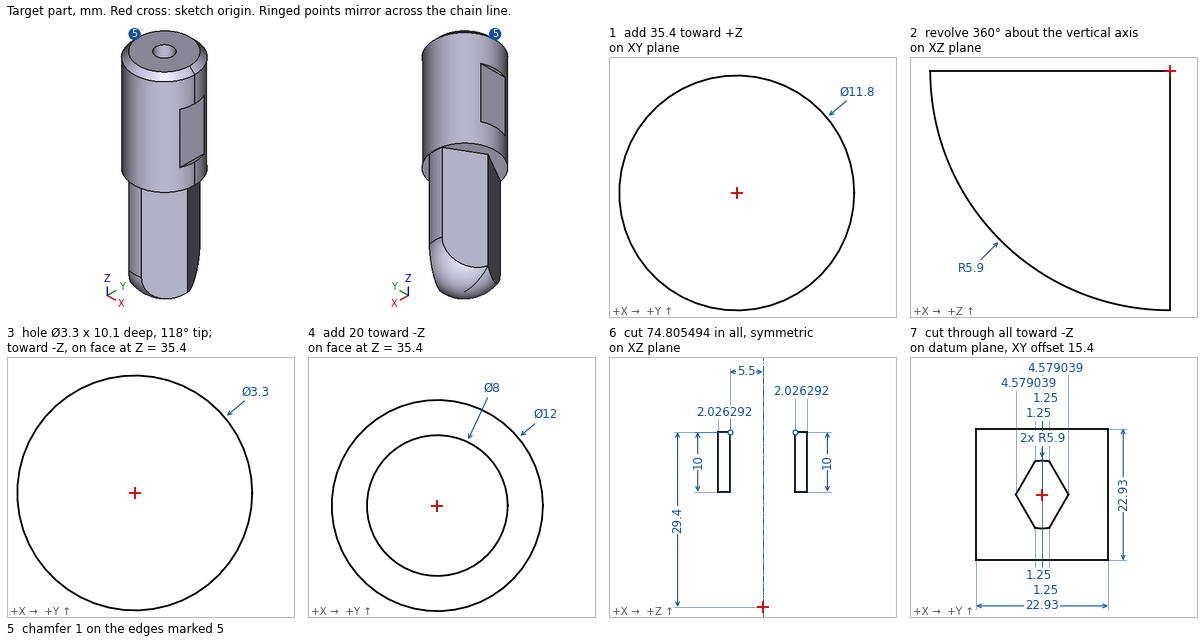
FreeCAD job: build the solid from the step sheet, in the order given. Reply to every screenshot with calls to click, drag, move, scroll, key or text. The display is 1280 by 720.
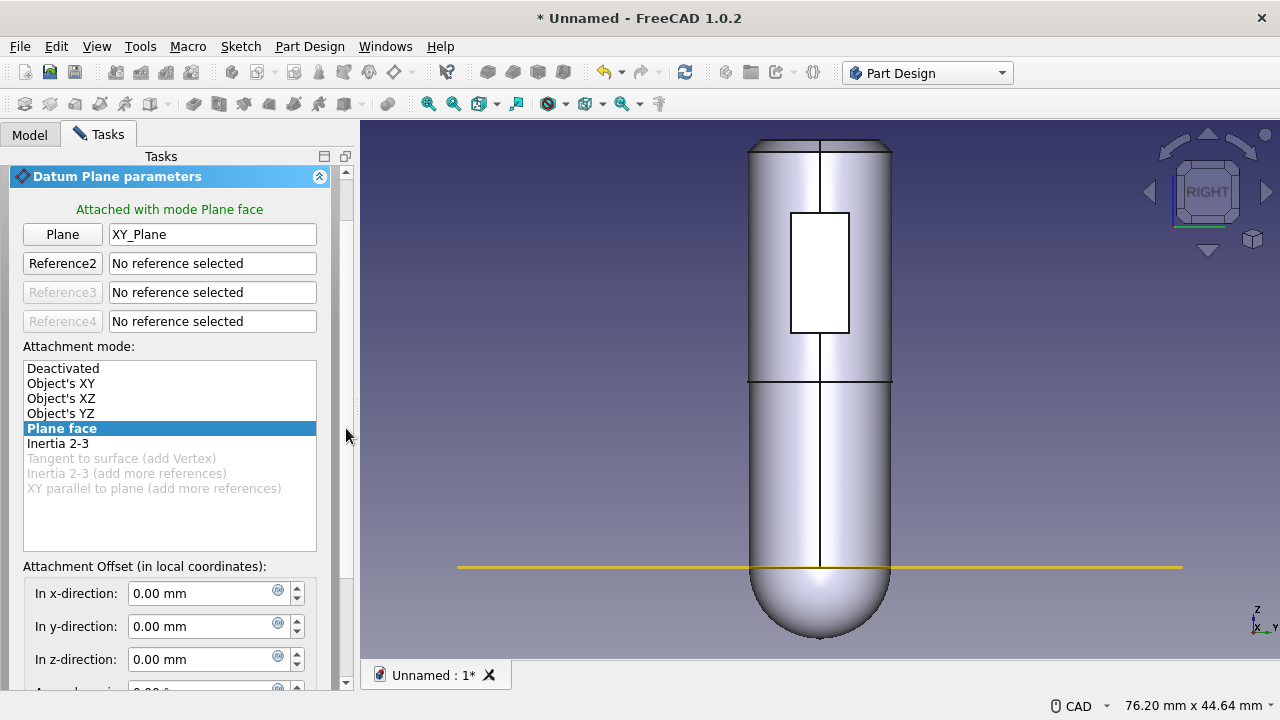
triple_click(210, 600)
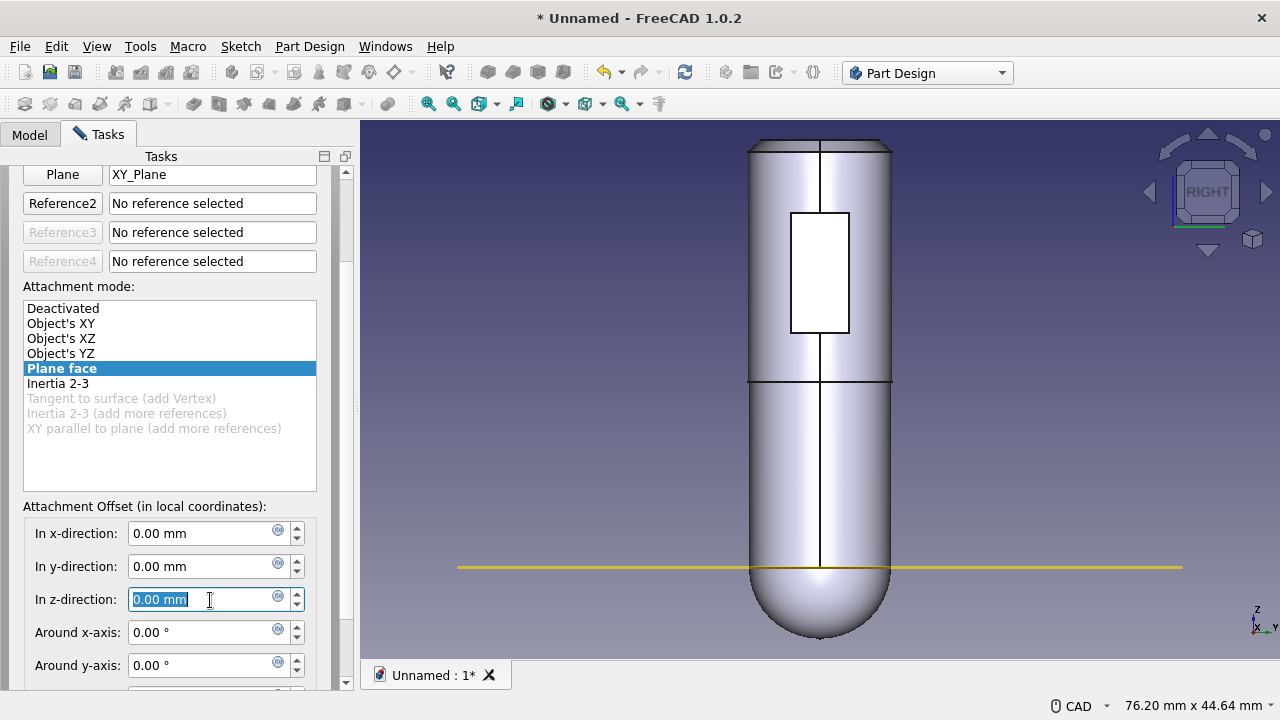
text(15.4)
key(Tab)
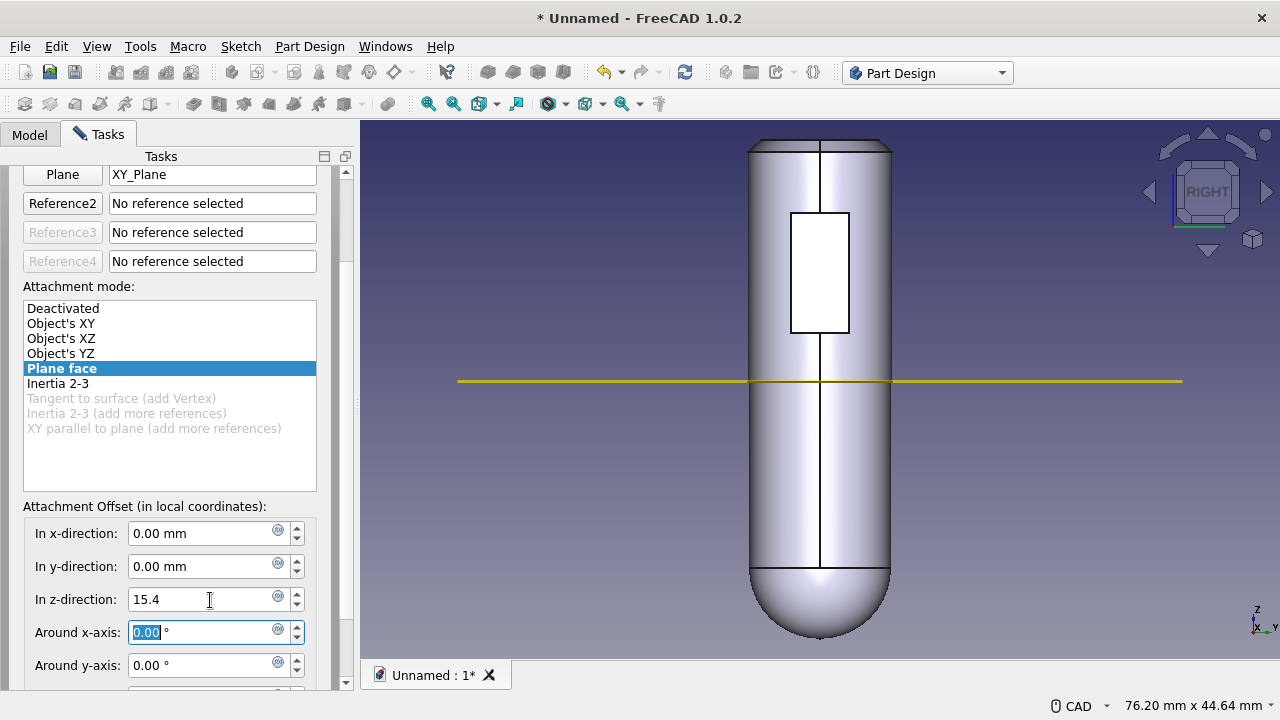
scroll(346, 428, up, 3)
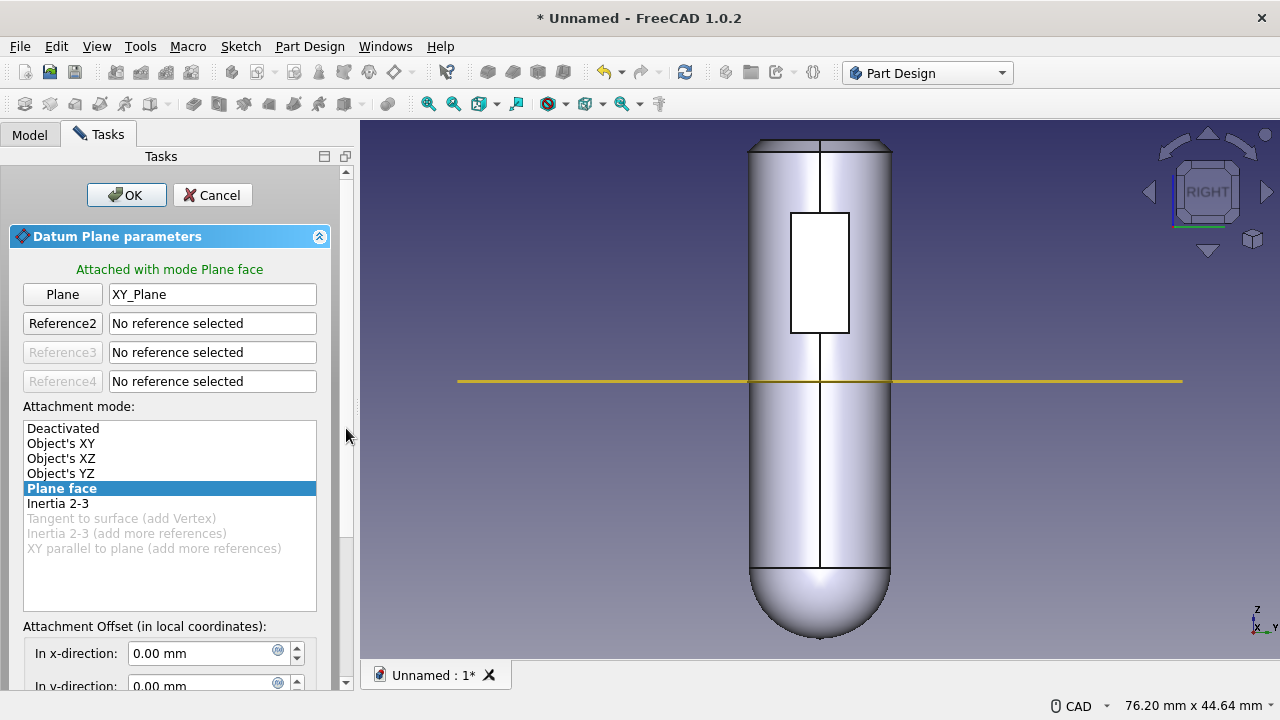
click(127, 195)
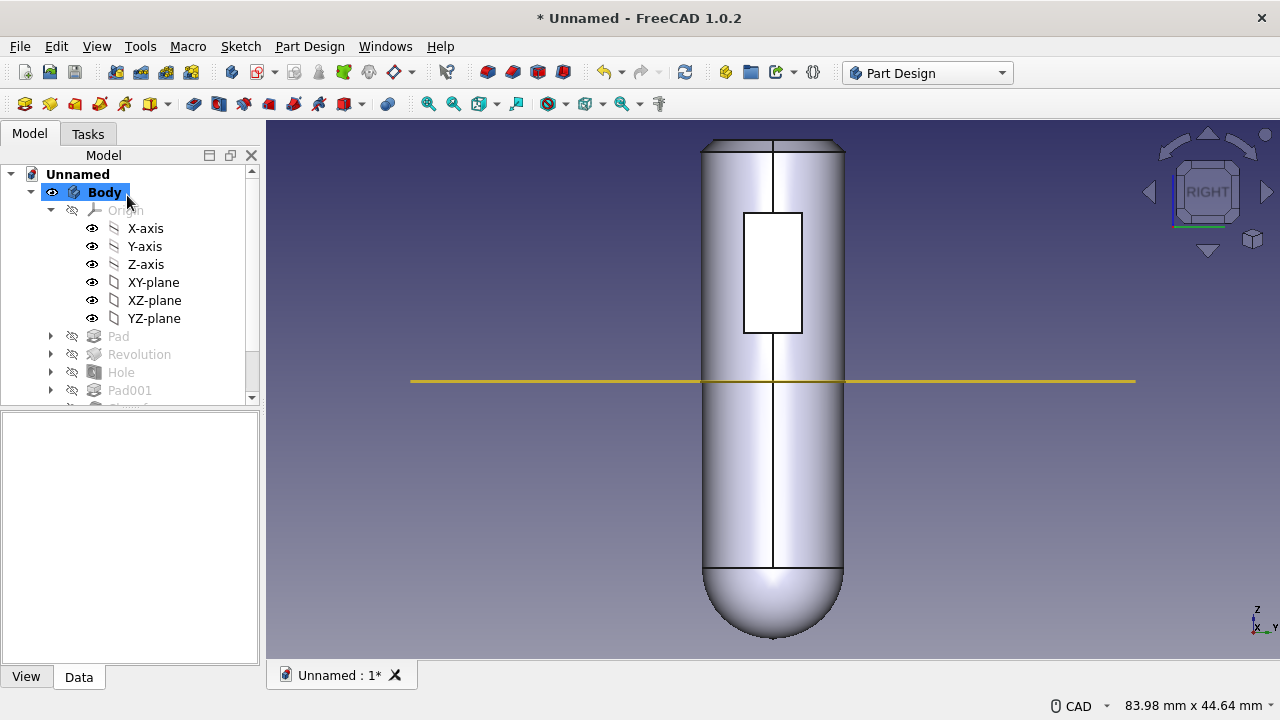
scroll(101, 278, down, 3)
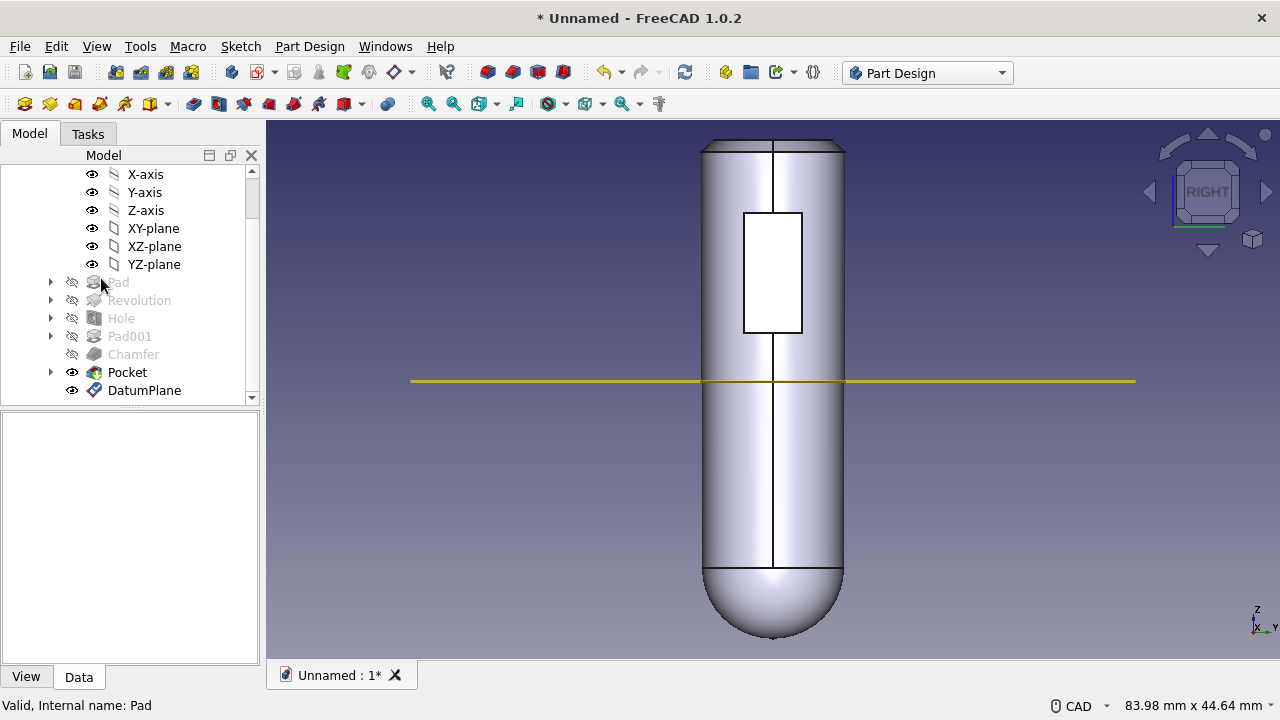
click(117, 390)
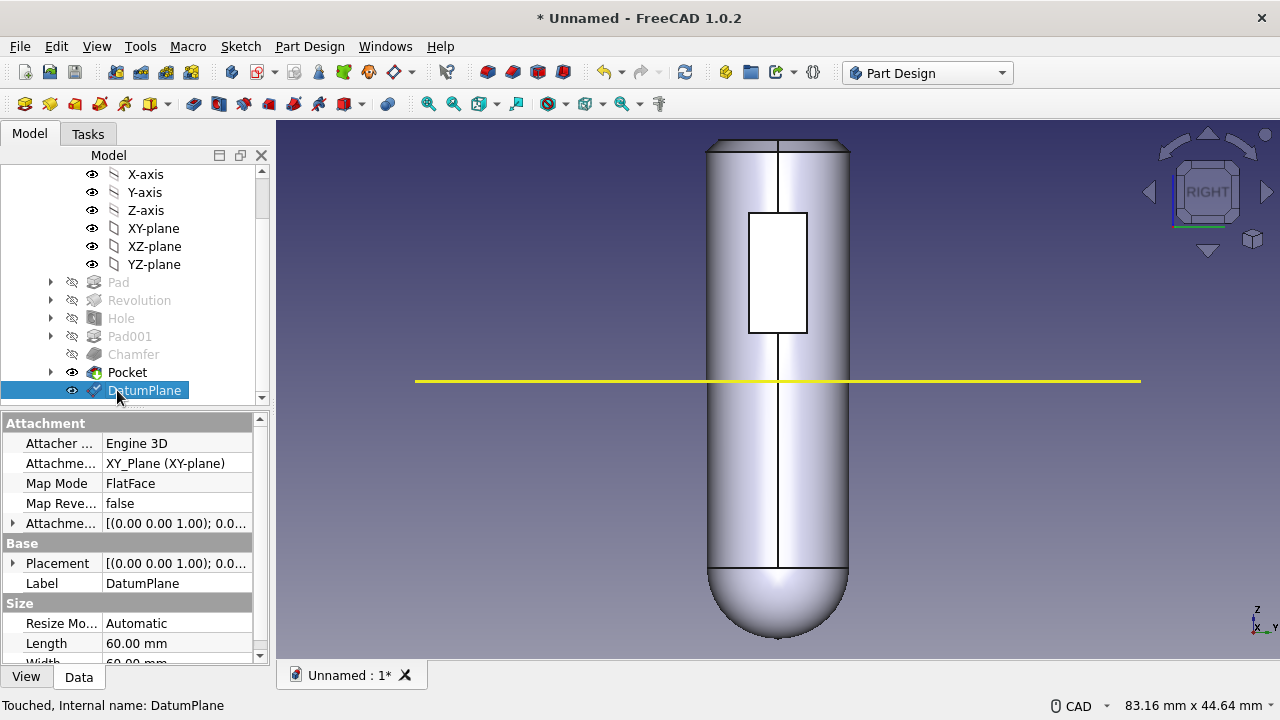
click(256, 72)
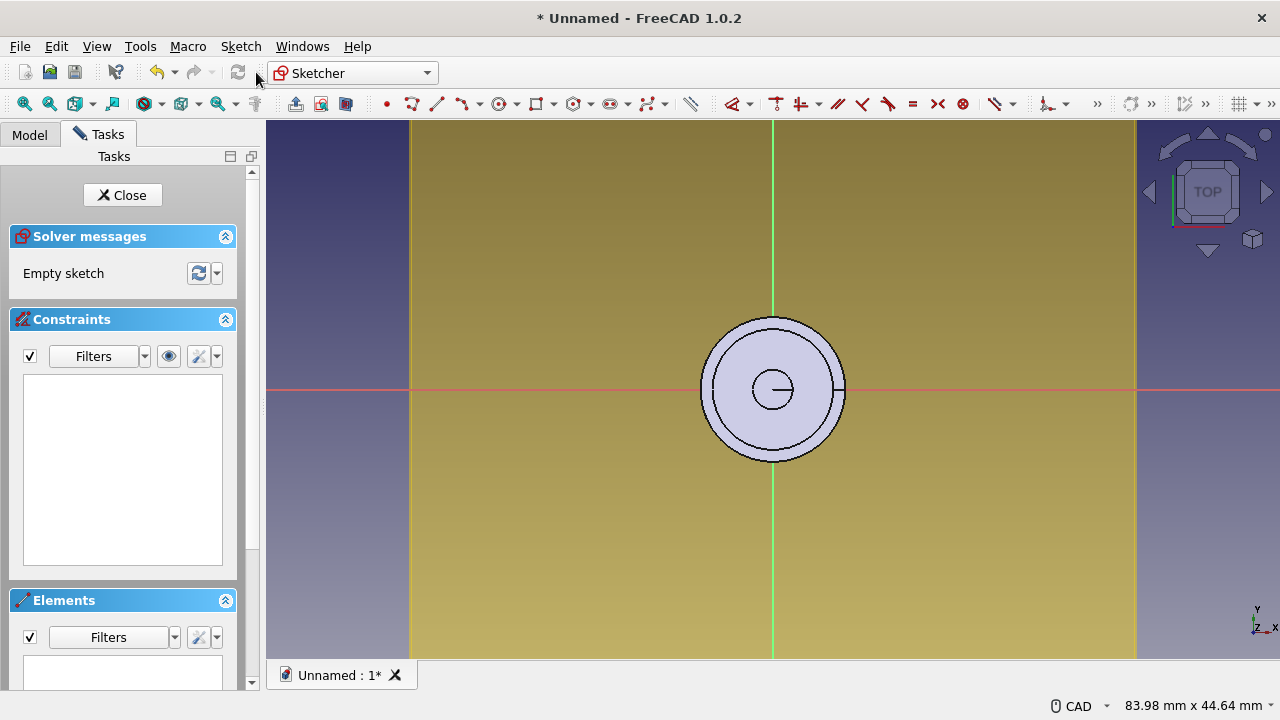
click(346, 104)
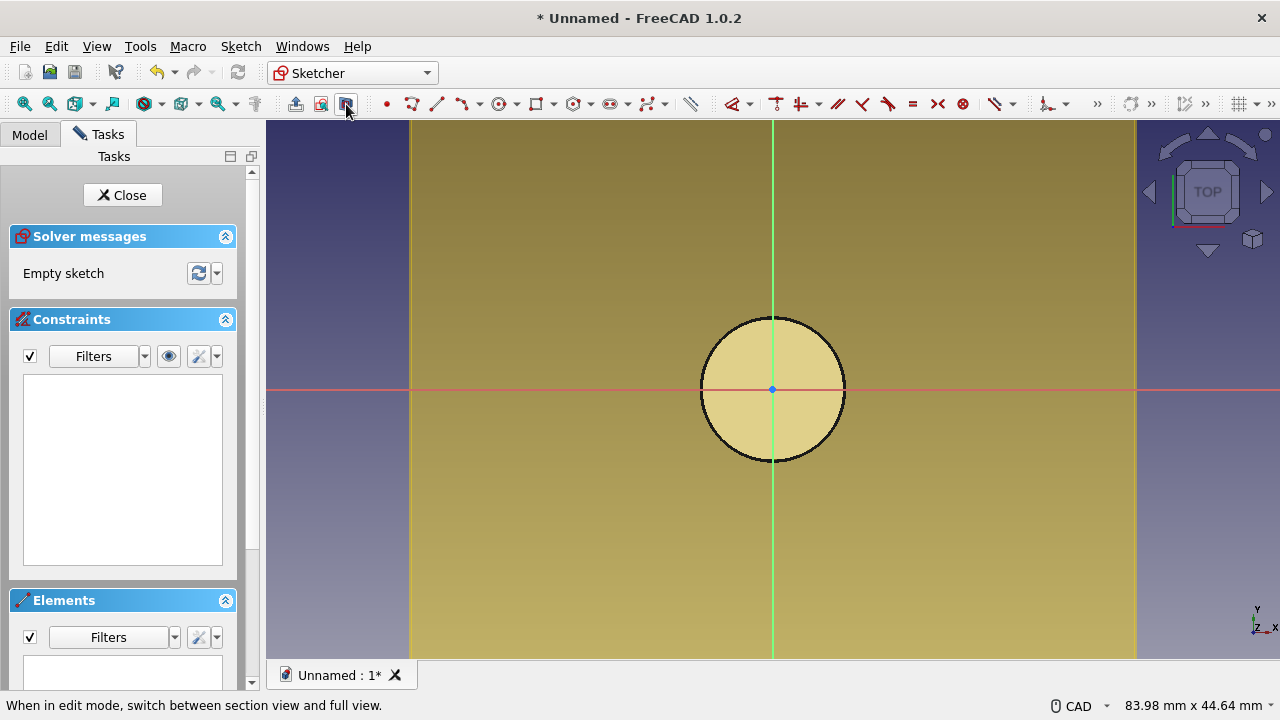
click(554, 104)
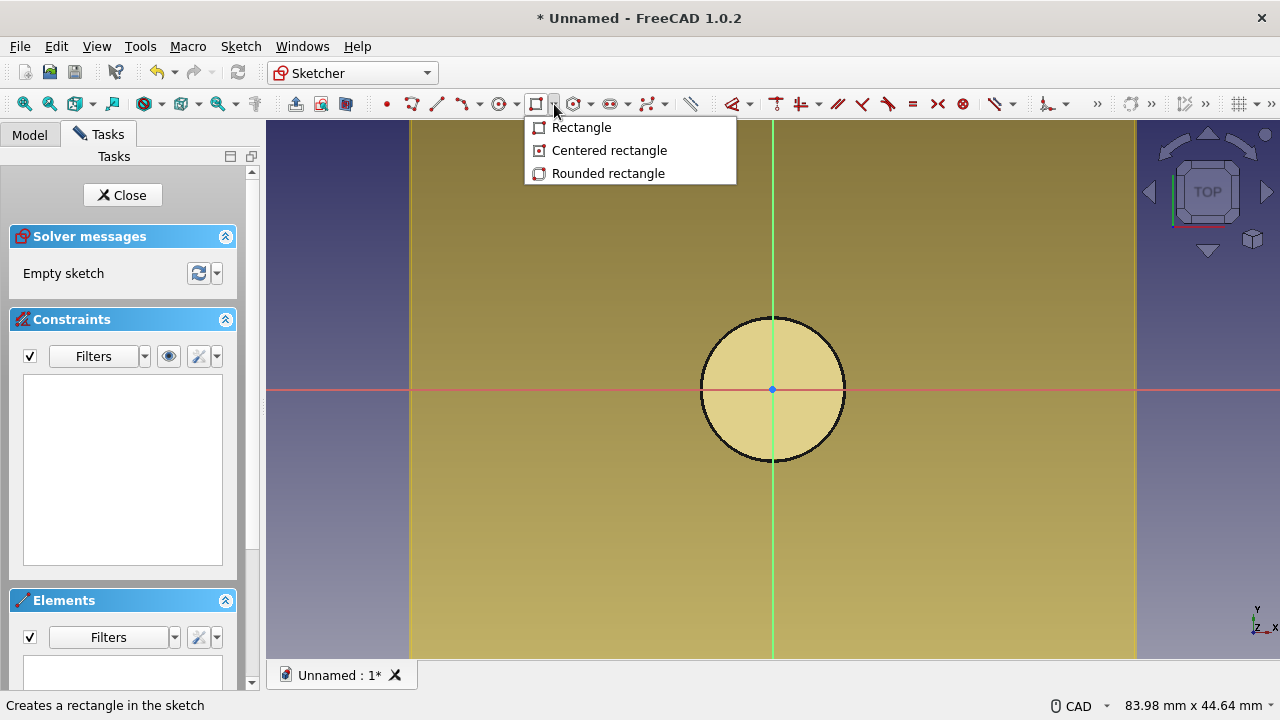
click(630, 150)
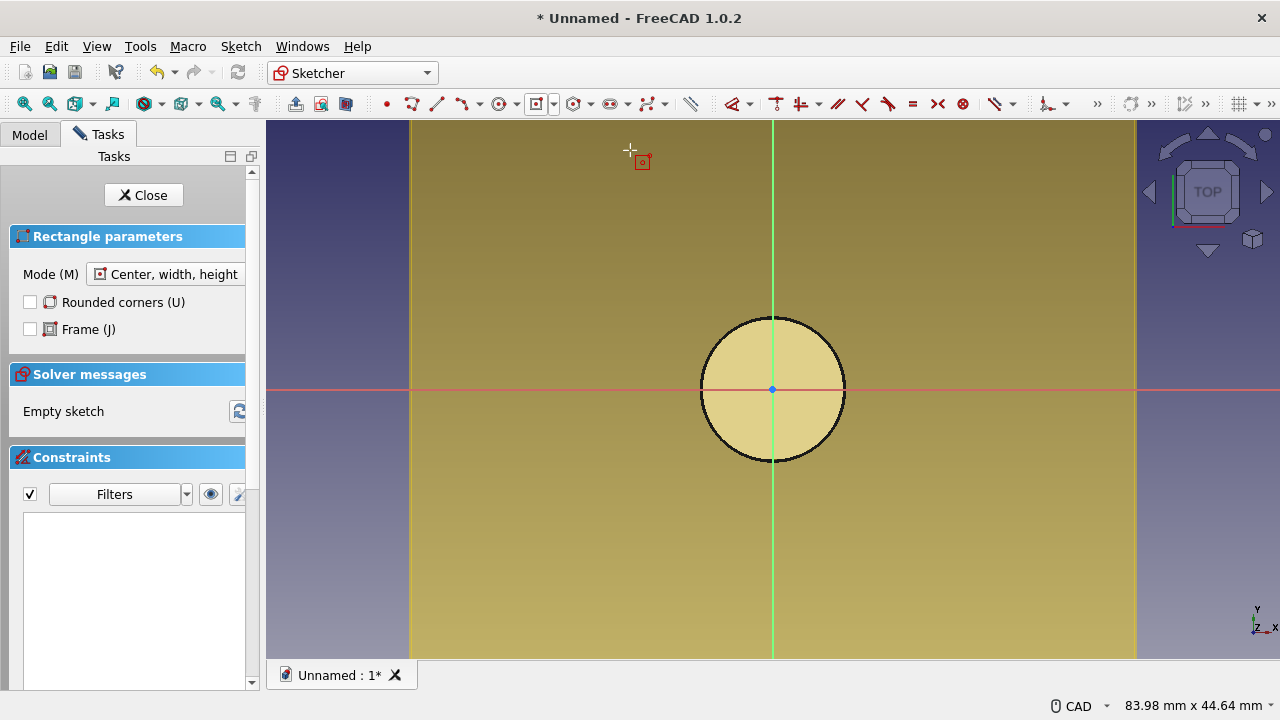
click(773, 390)
move(911, 251)